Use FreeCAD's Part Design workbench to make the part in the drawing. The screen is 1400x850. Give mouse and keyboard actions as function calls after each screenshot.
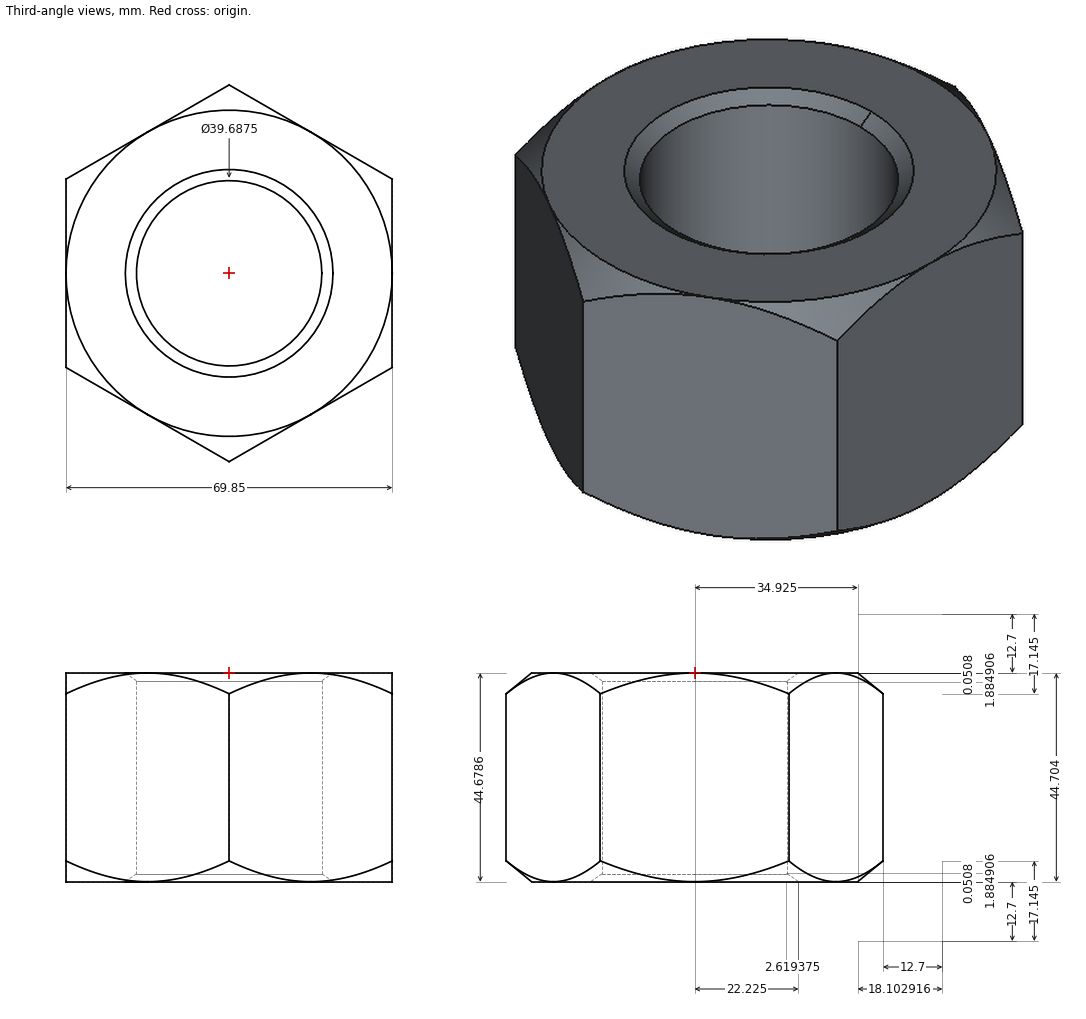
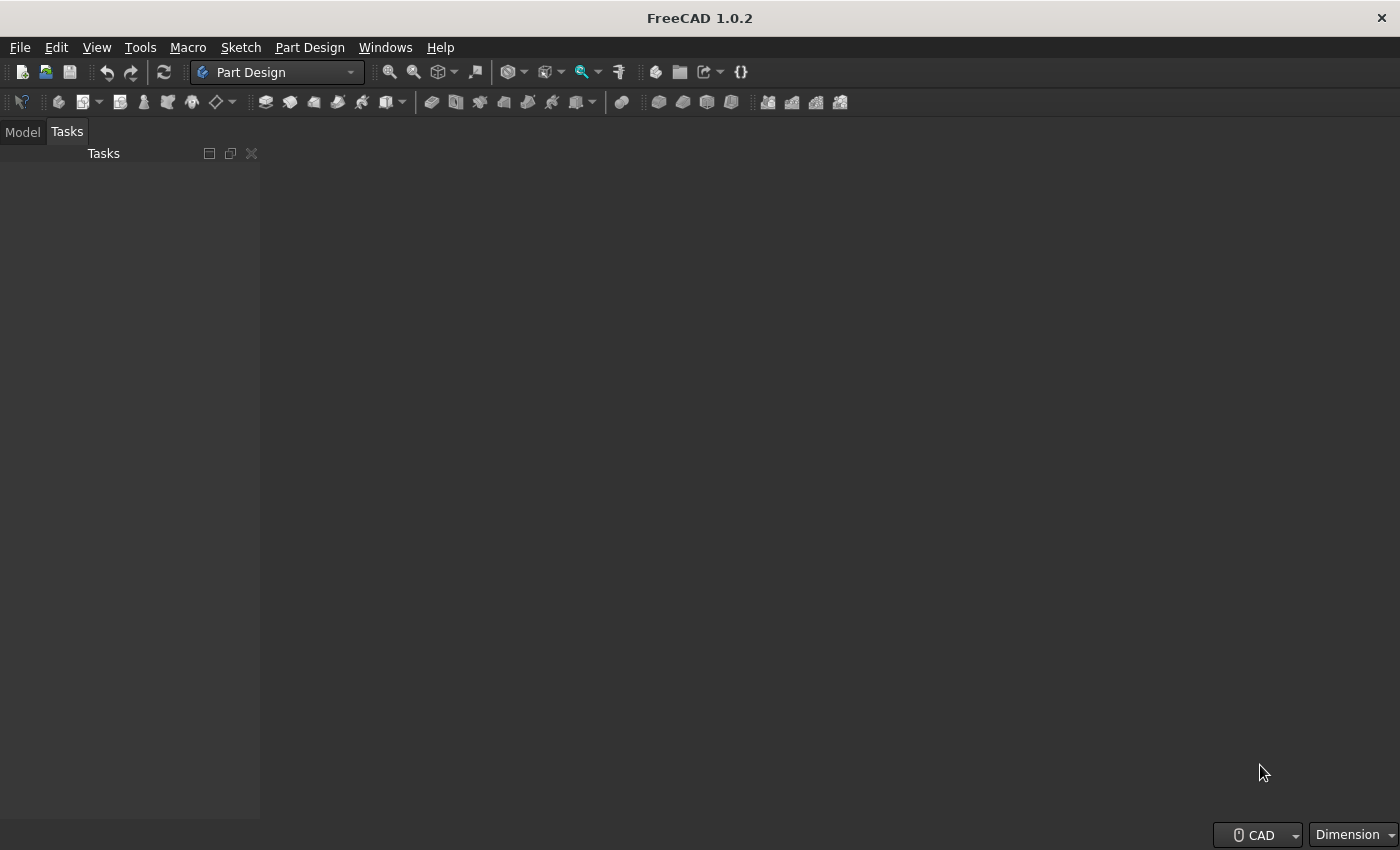
click(22, 72)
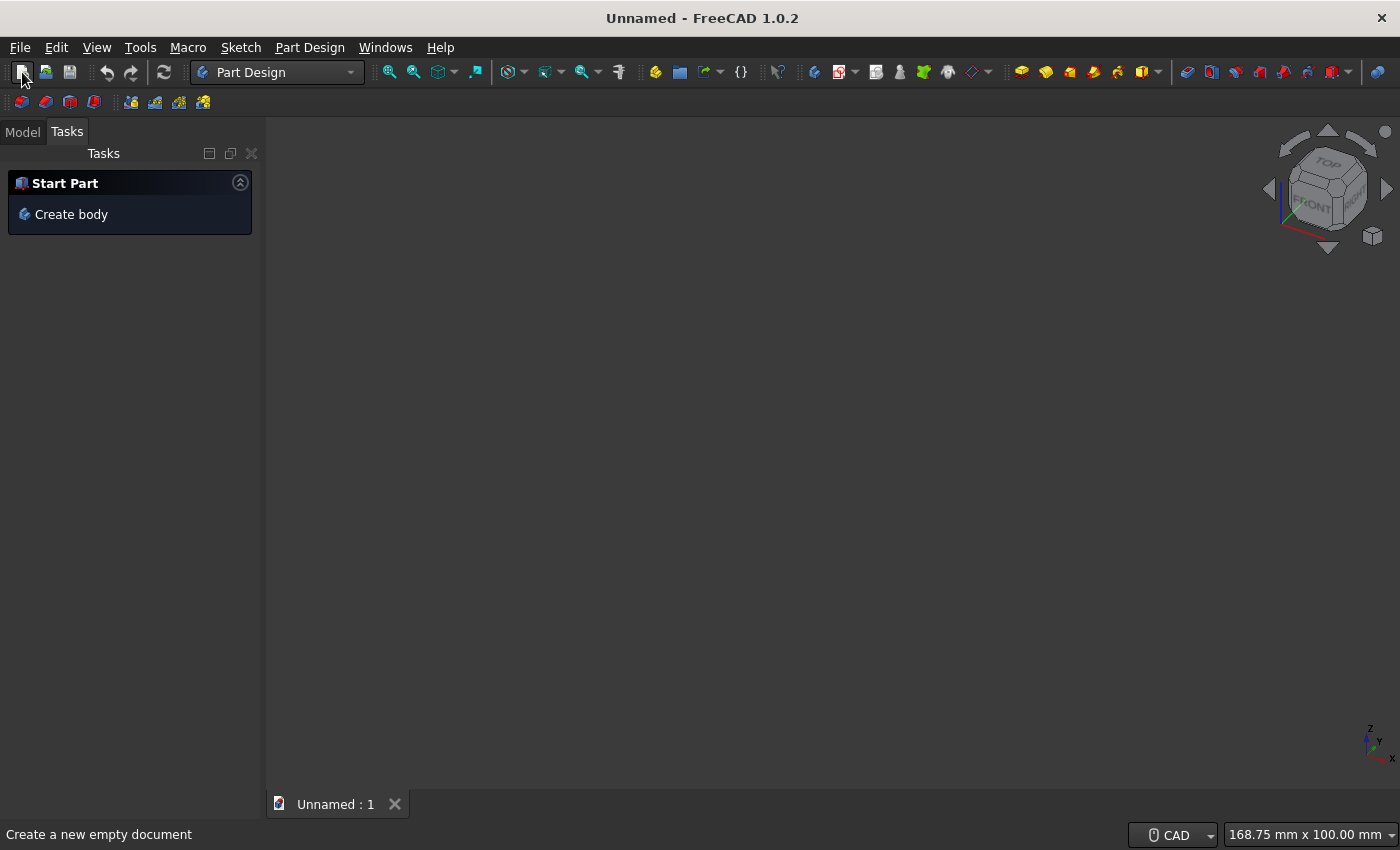
click(816, 72)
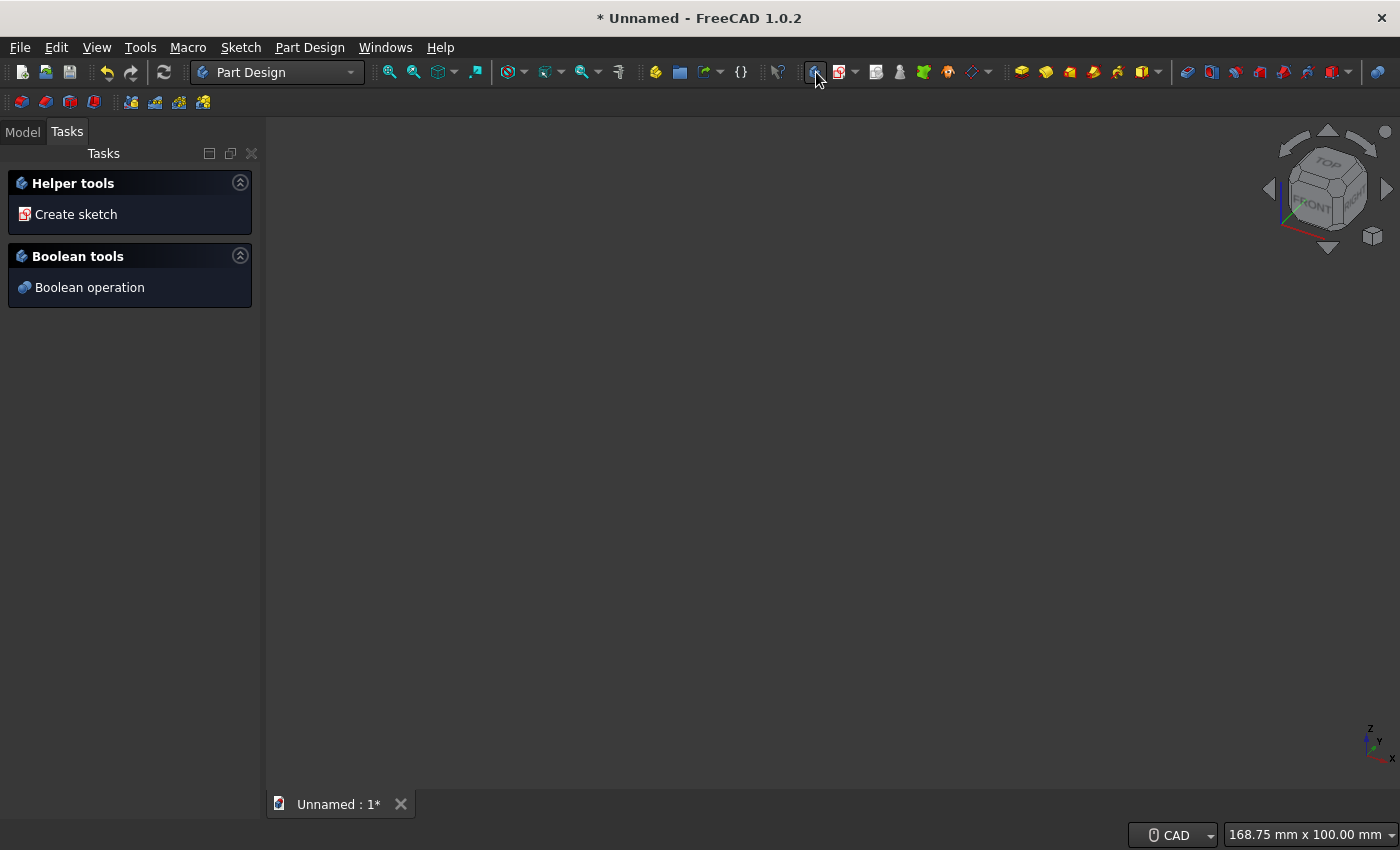
click(23, 131)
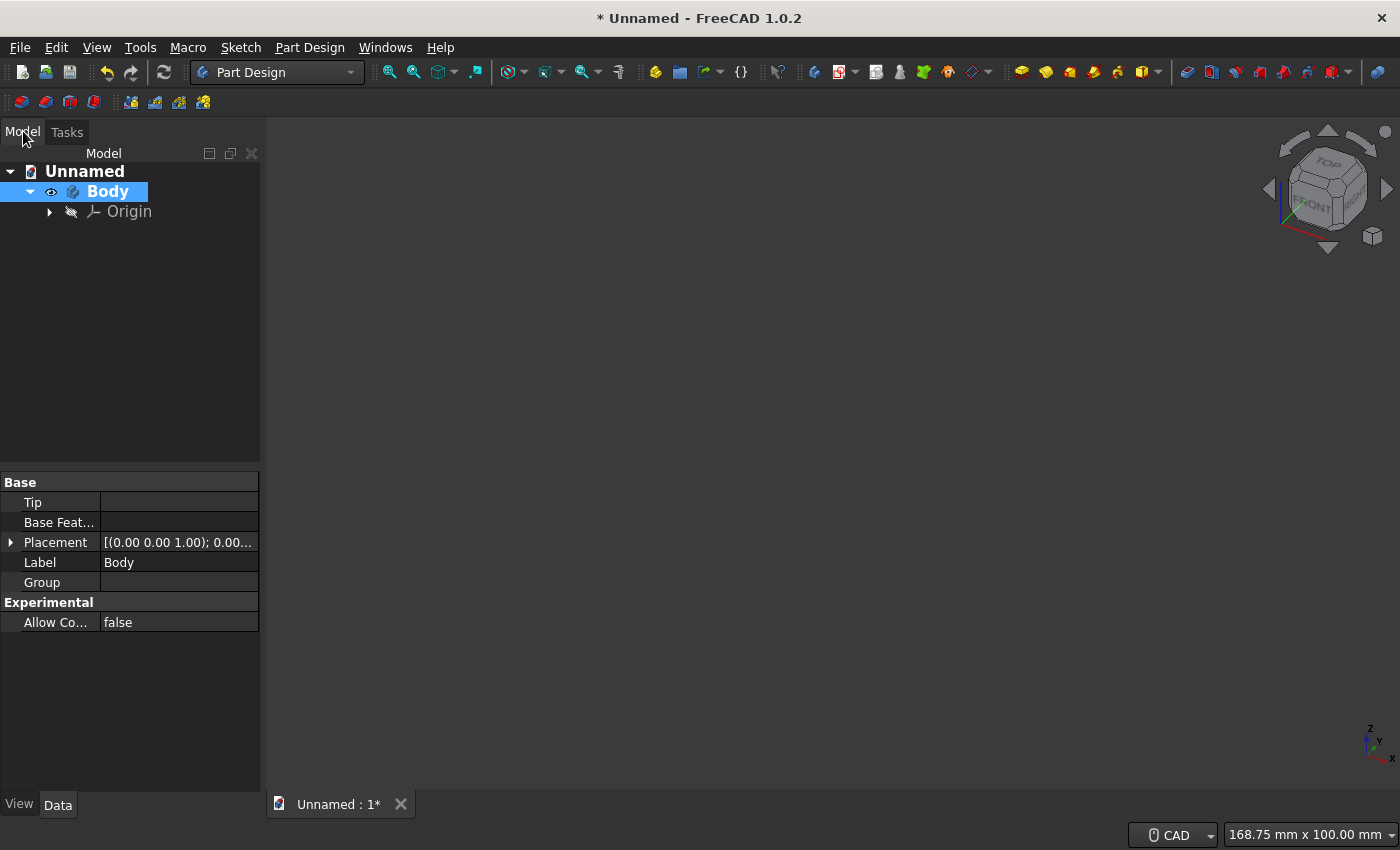
click(50, 212)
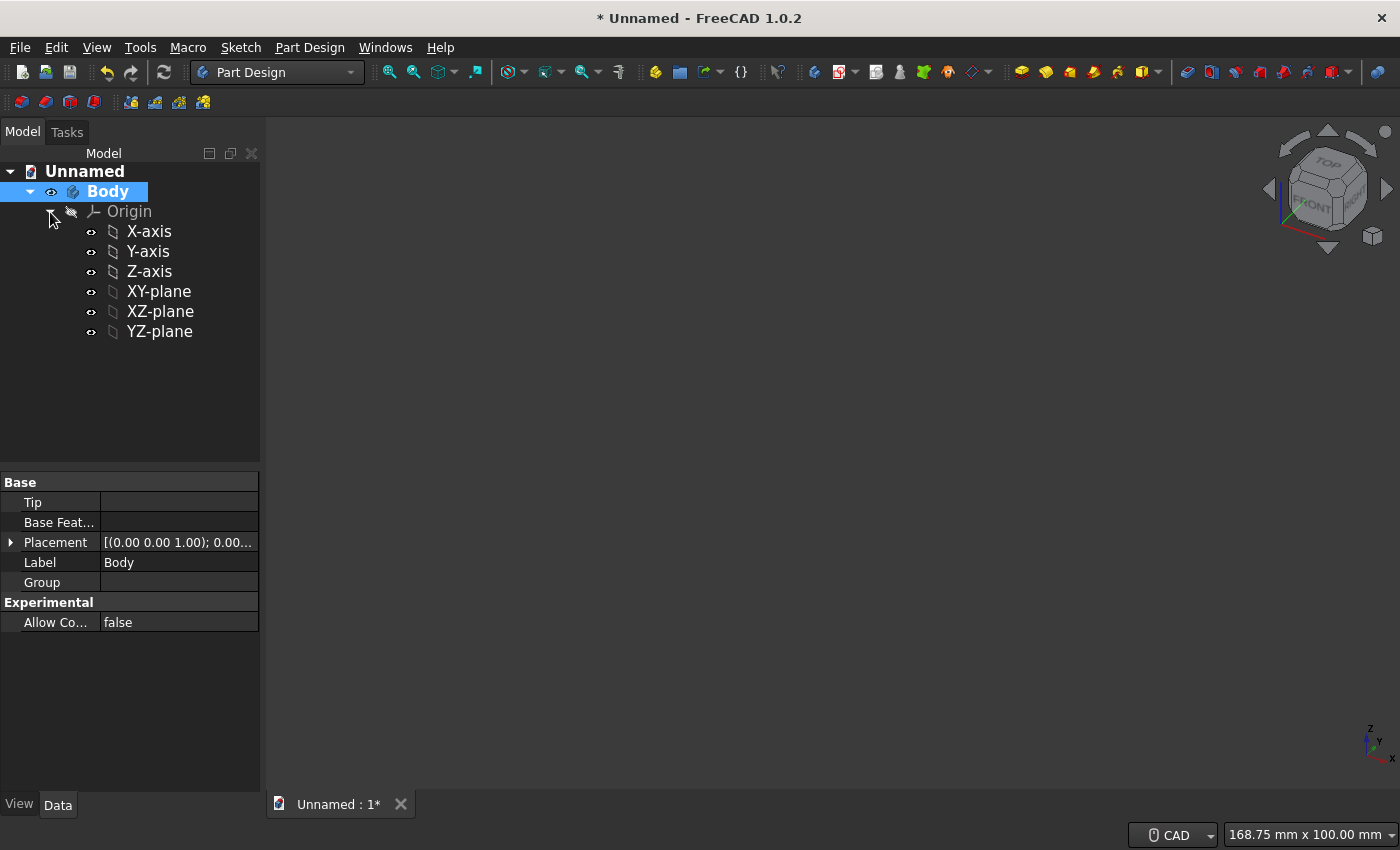
click(136, 292)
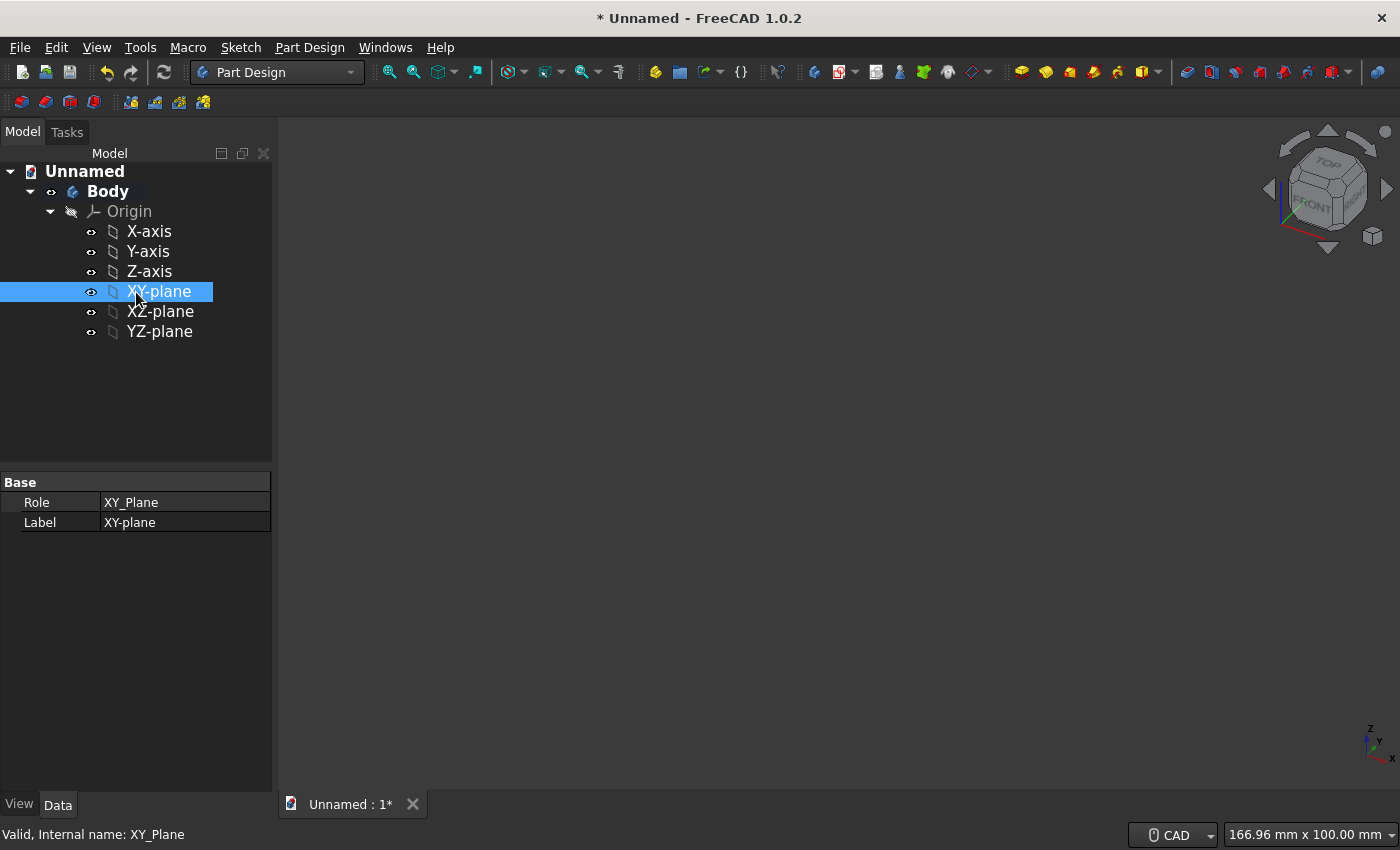
click(972, 72)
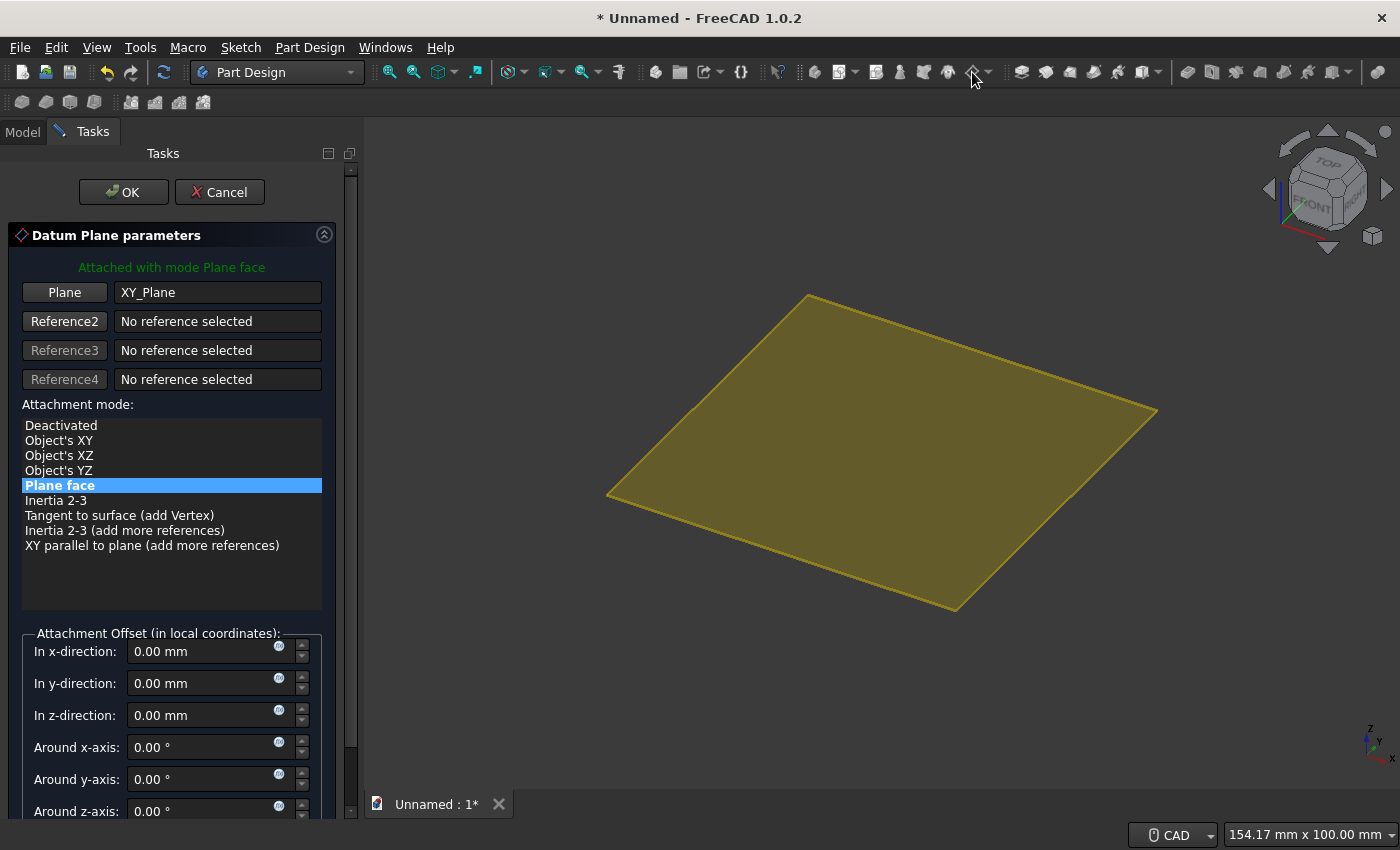
triple_click(210, 715)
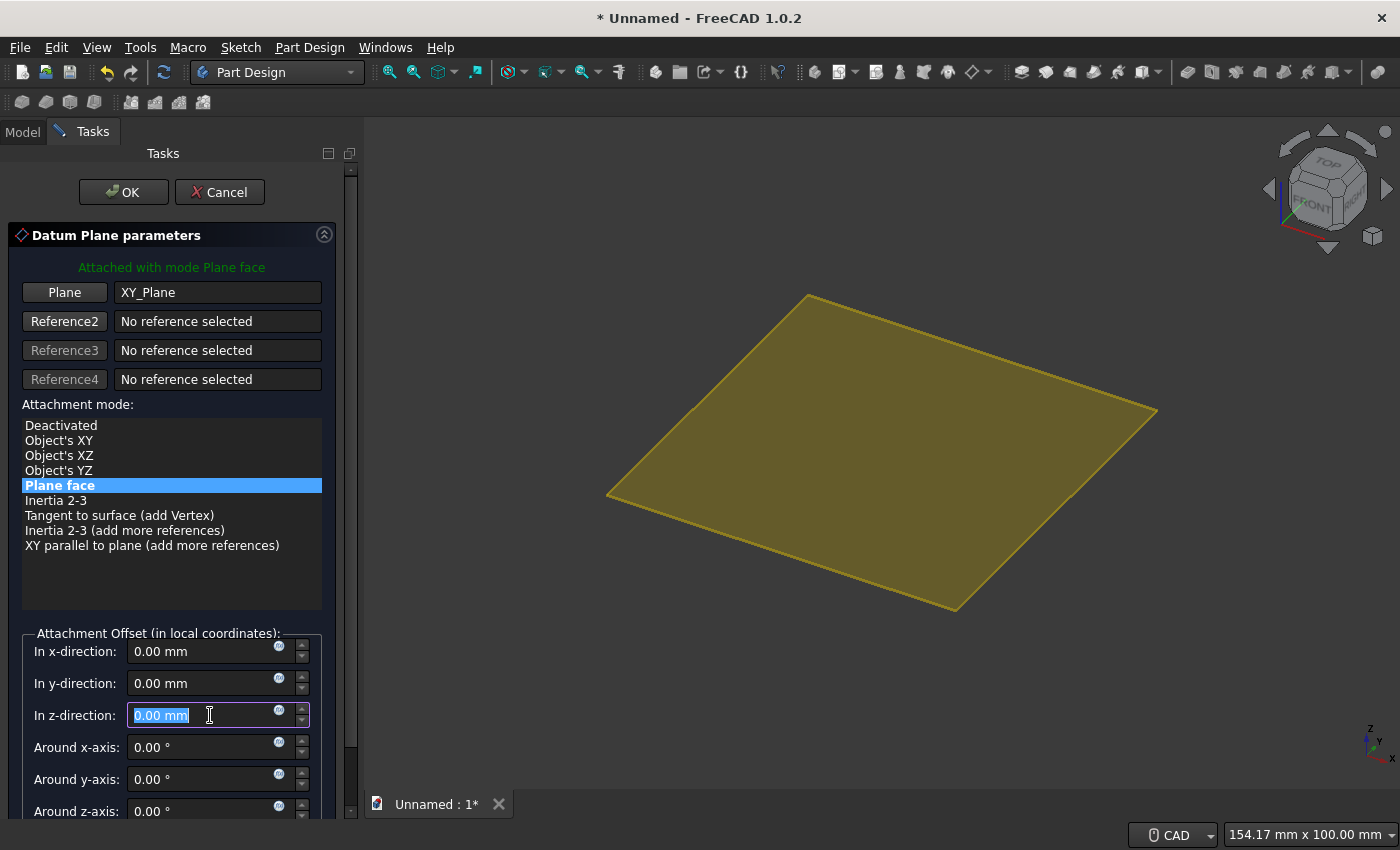
text(-44.6786)
key(Tab)